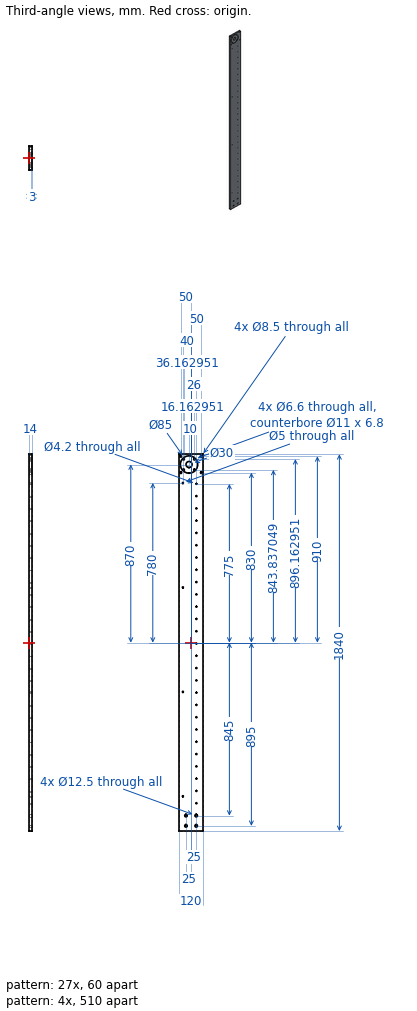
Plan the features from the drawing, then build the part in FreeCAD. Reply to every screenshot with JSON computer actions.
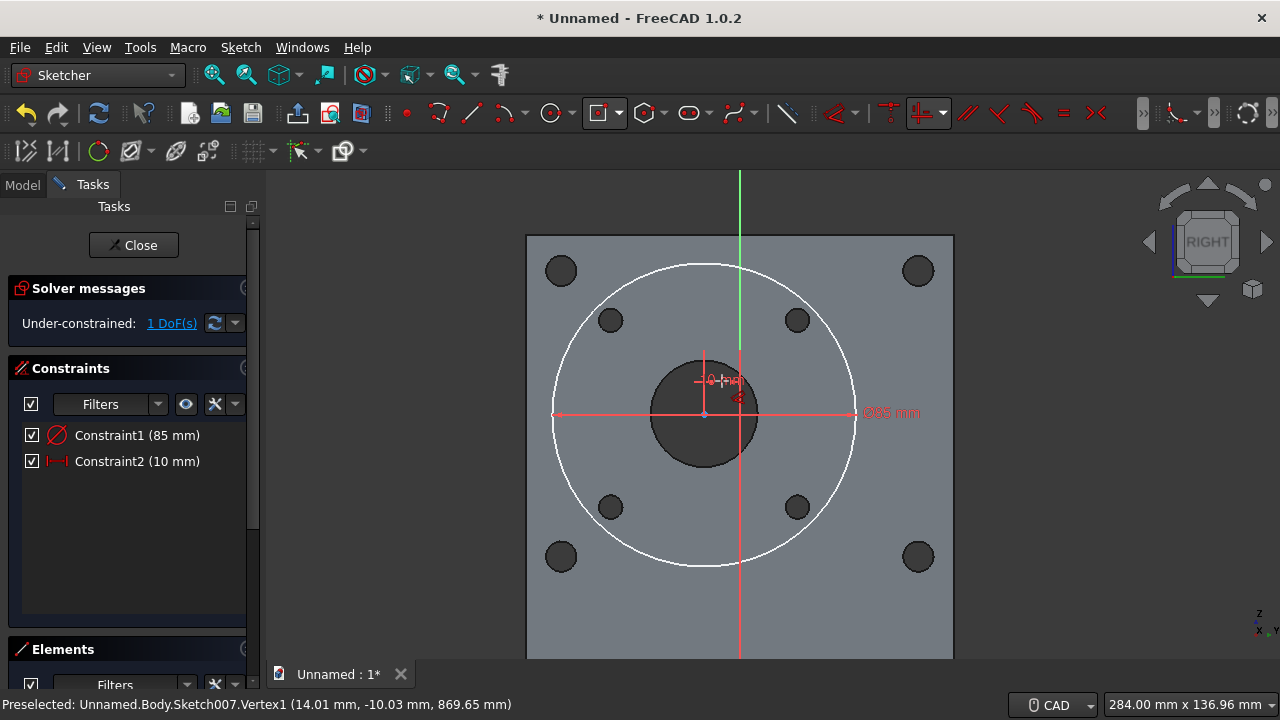
{"action": "left_click", "coordinate": [704, 415]}
{"action": "left_click", "coordinate": [774, 523]}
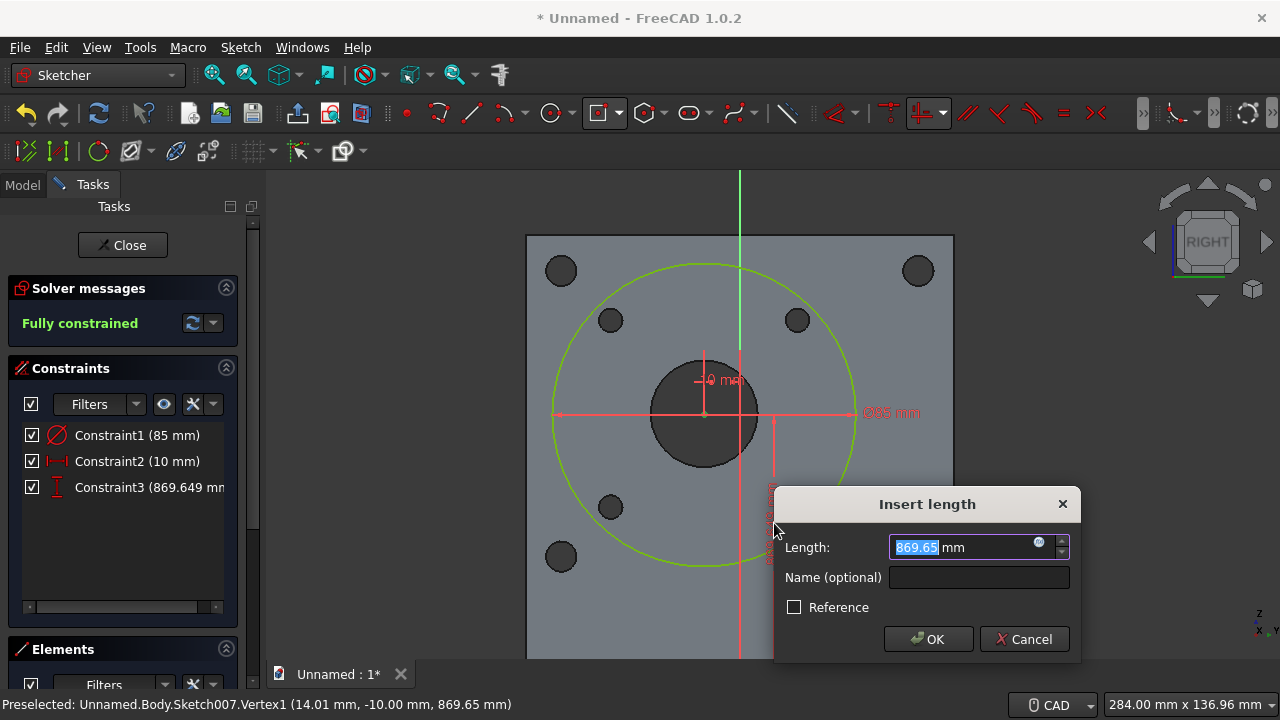
{"action": "type", "text": "870"}
{"action": "key", "text": "Return"}
{"action": "key", "text": "Escape"}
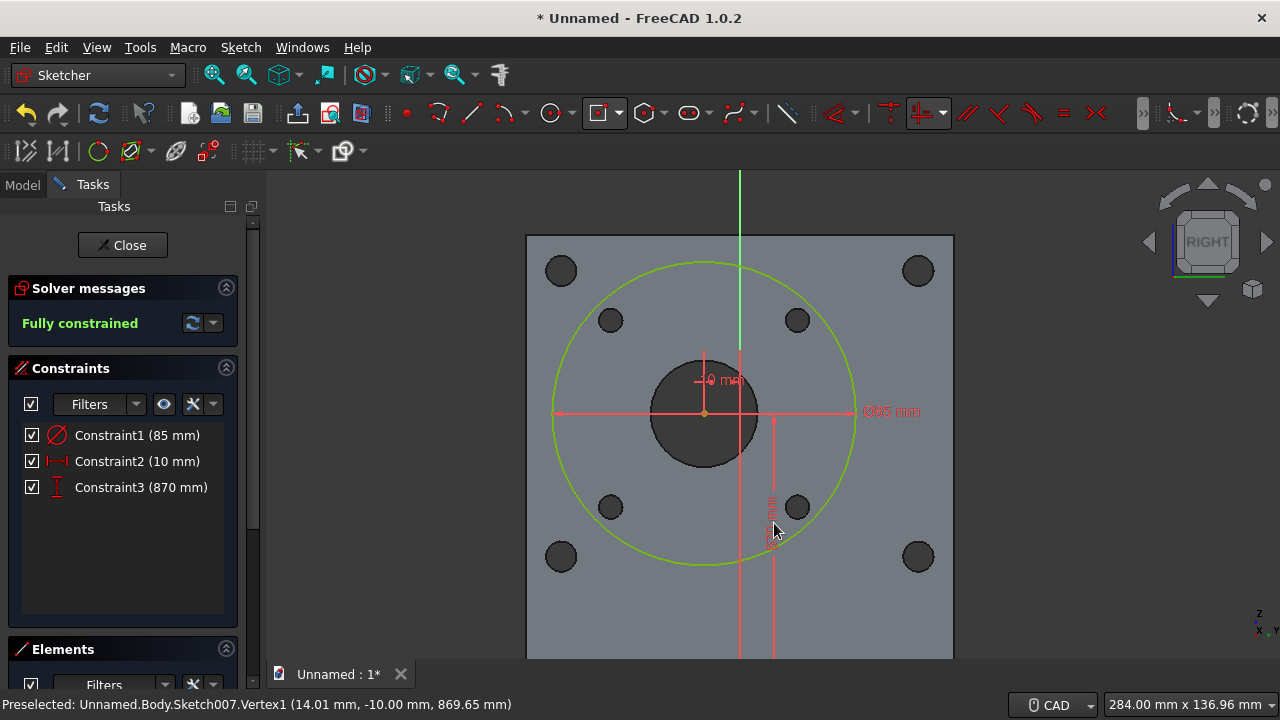
{"action": "left_click", "coordinate": [123, 245]}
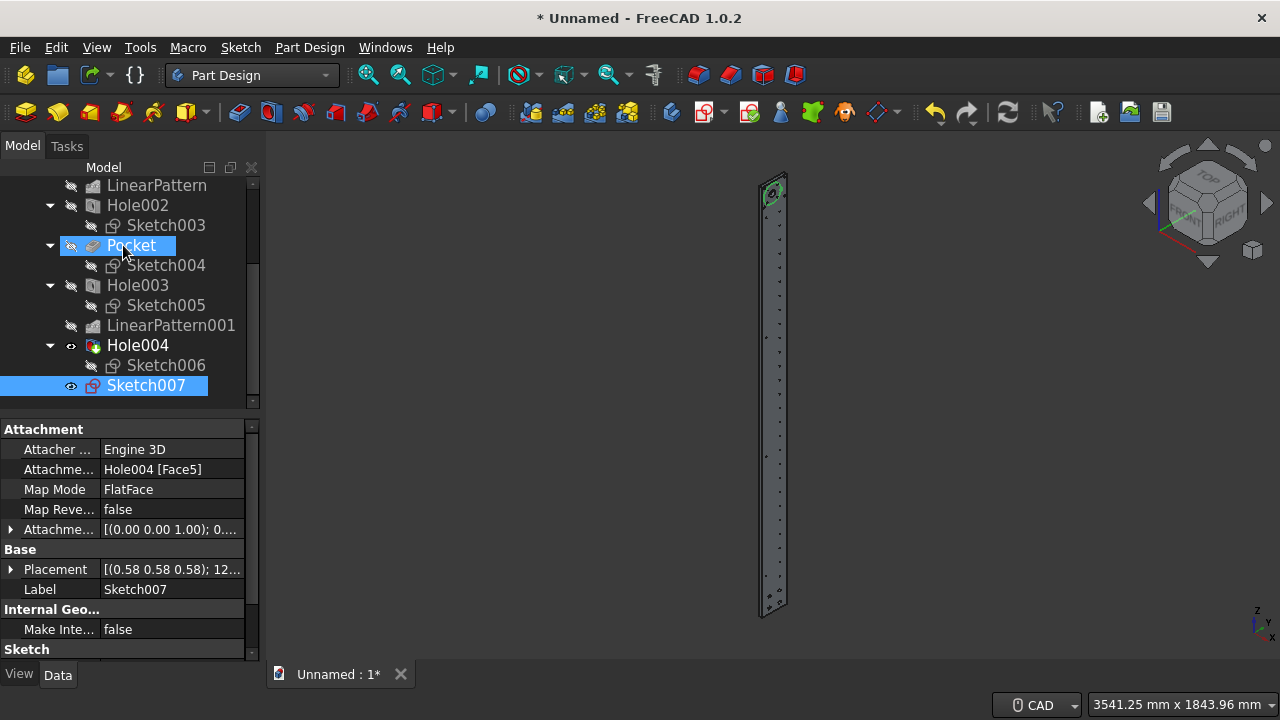
{"action": "left_click", "coordinate": [240, 112]}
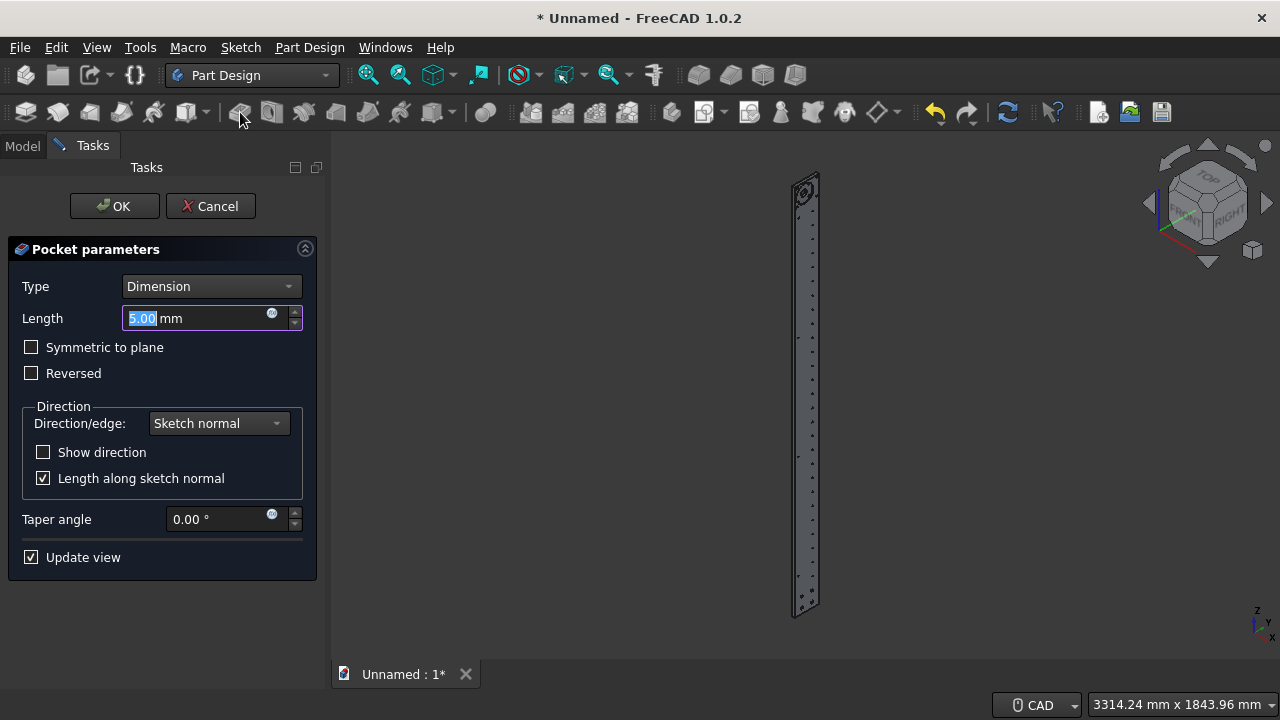
{"action": "type", "text": "3"}
{"action": "key", "text": "Tab"}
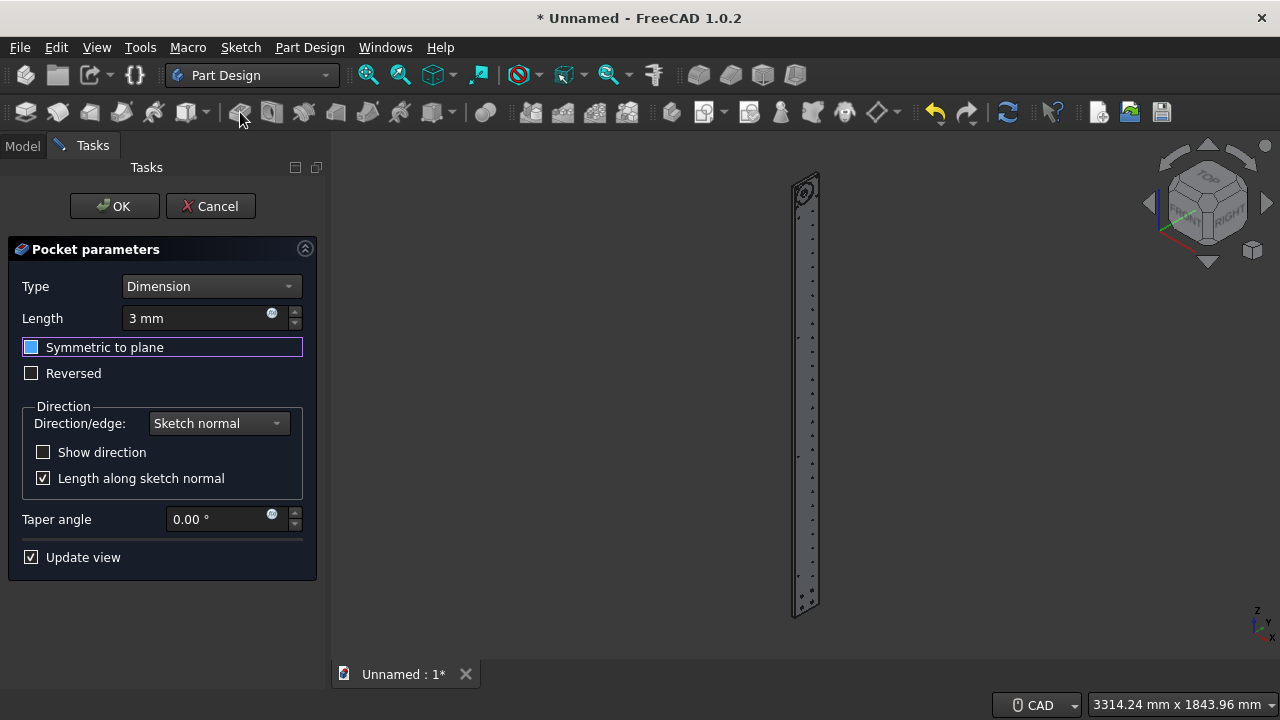
{"action": "left_click", "coordinate": [115, 206]}